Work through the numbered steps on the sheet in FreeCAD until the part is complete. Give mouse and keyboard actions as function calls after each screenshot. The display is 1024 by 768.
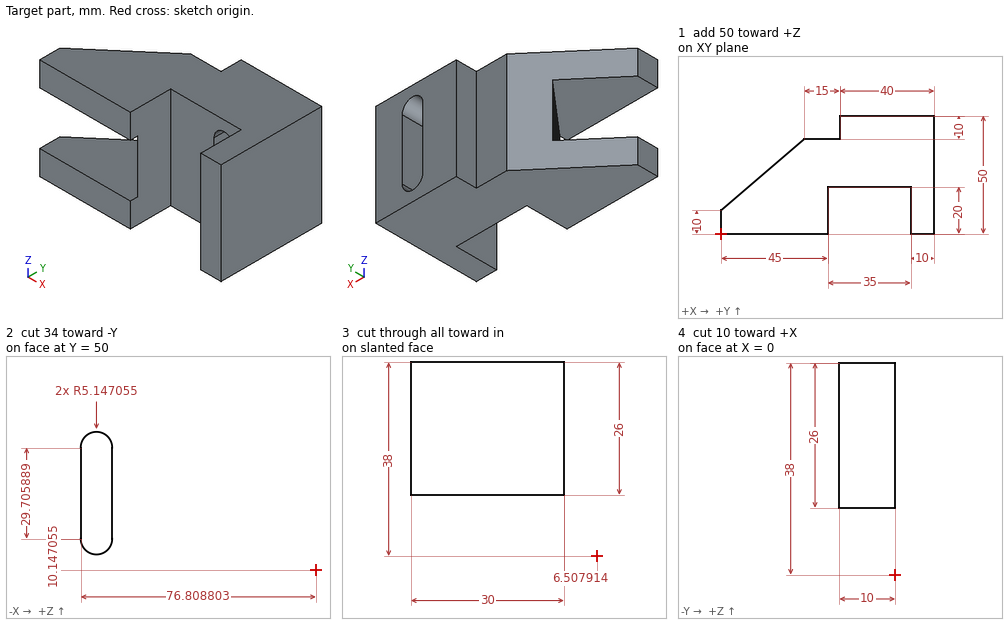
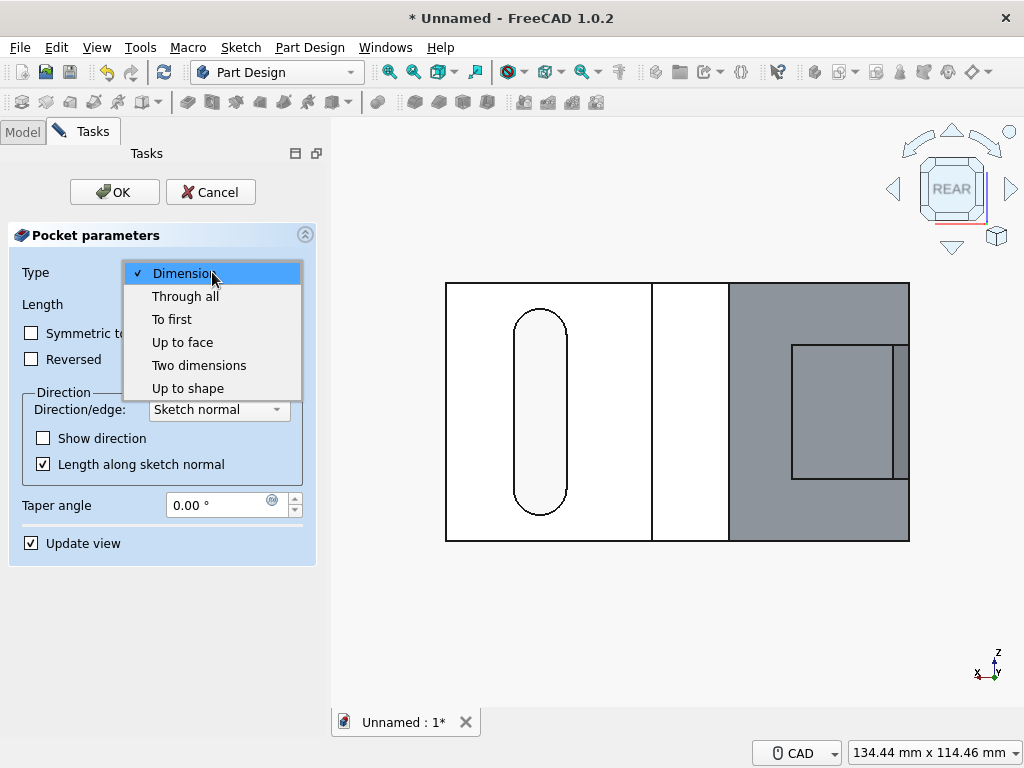
click(212, 296)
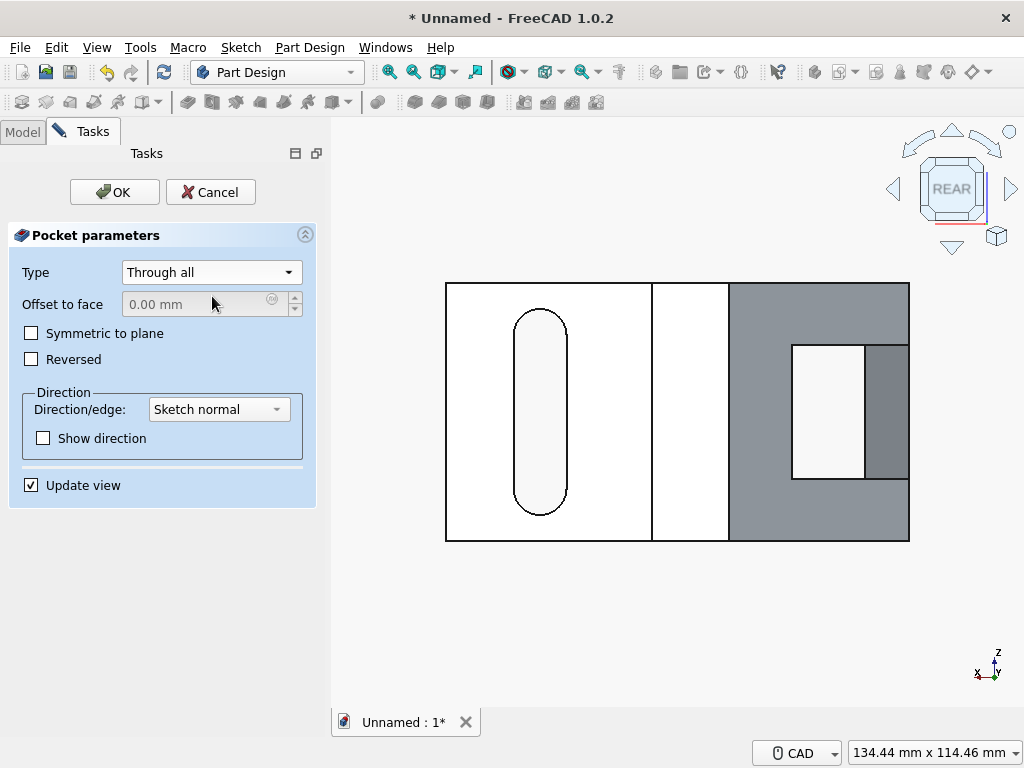
click(115, 192)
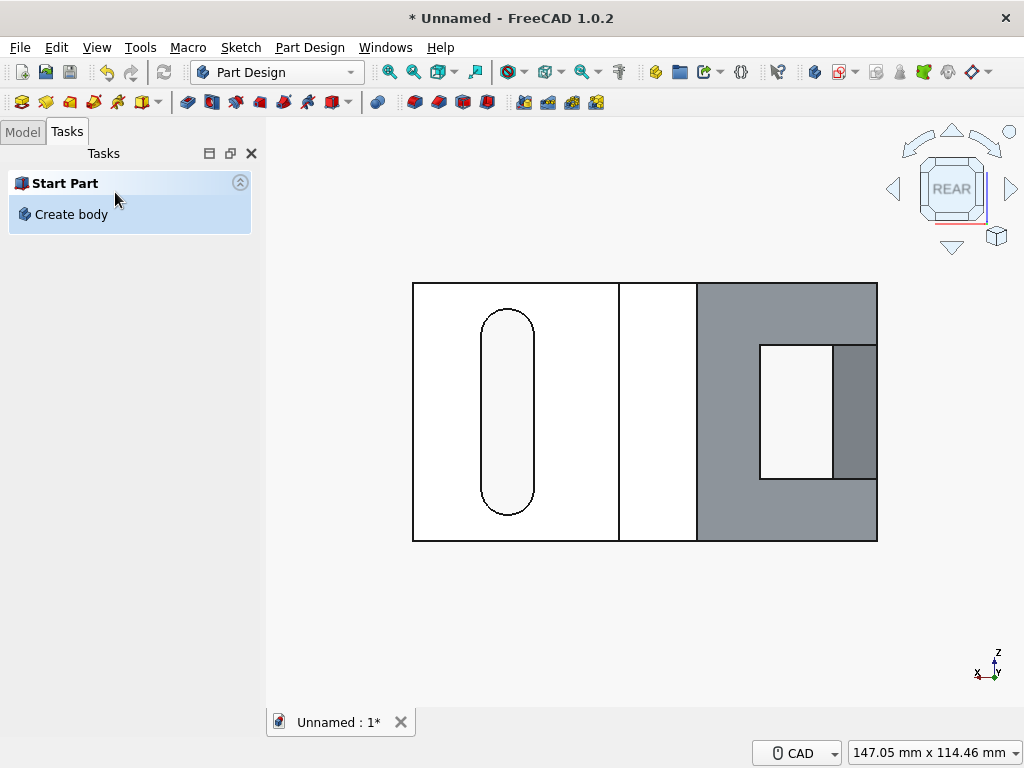
key(6)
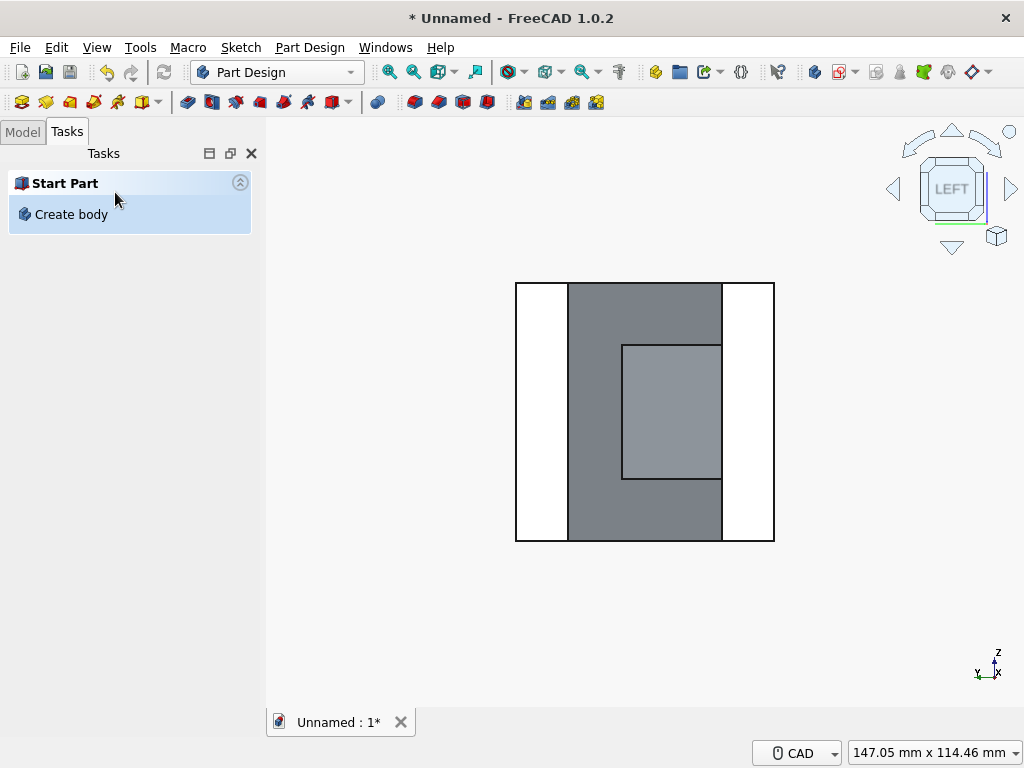
click(390, 72)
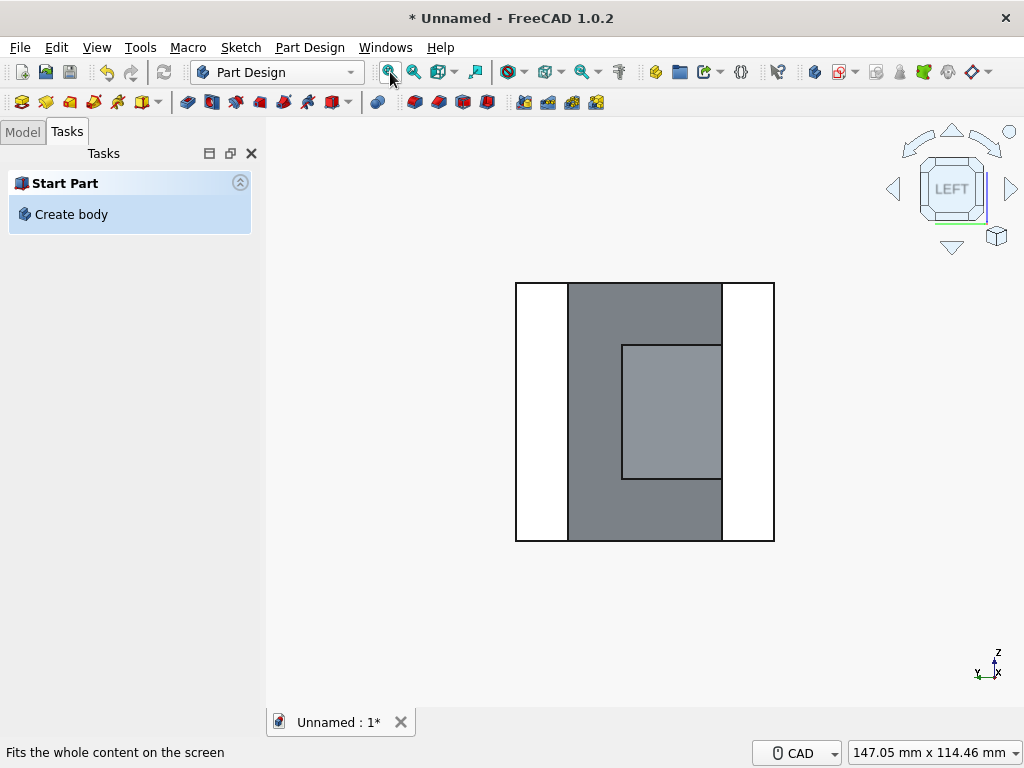
click(748, 337)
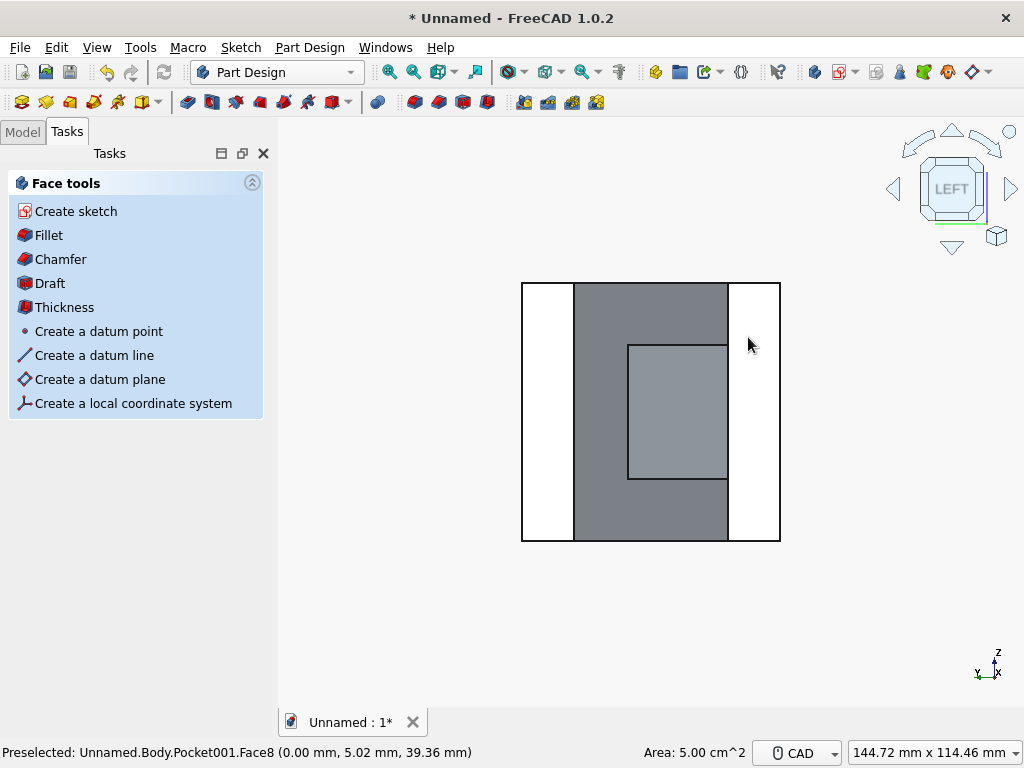
click(840, 72)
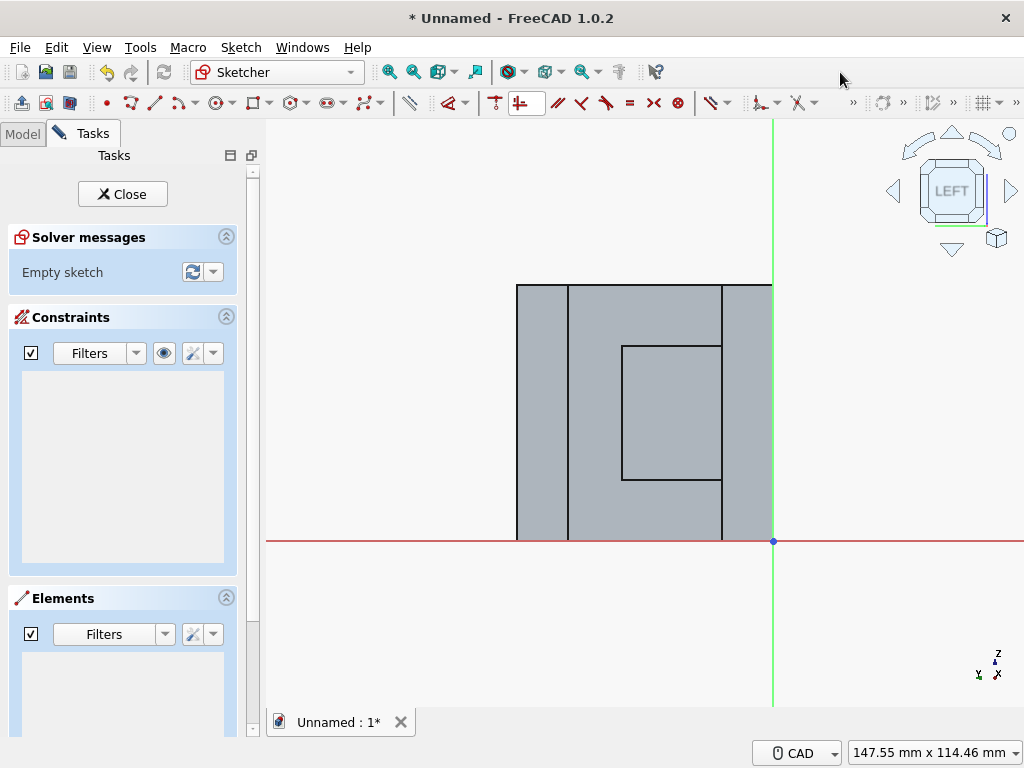
scroll(859, 481, up, 3)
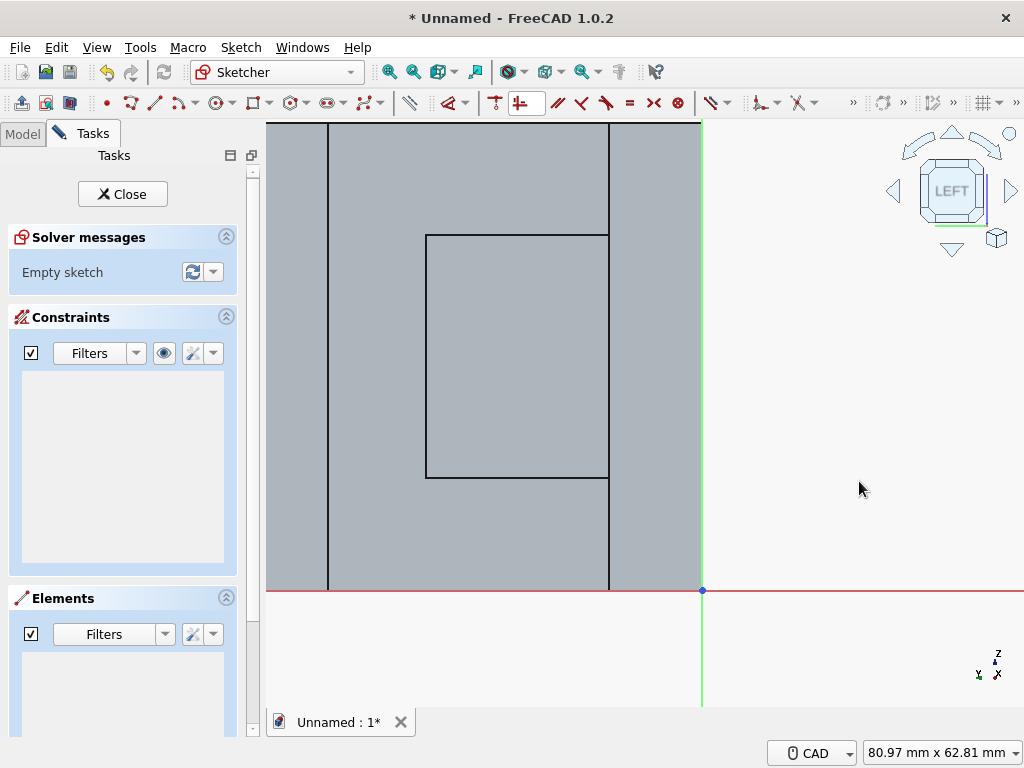
click(254, 104)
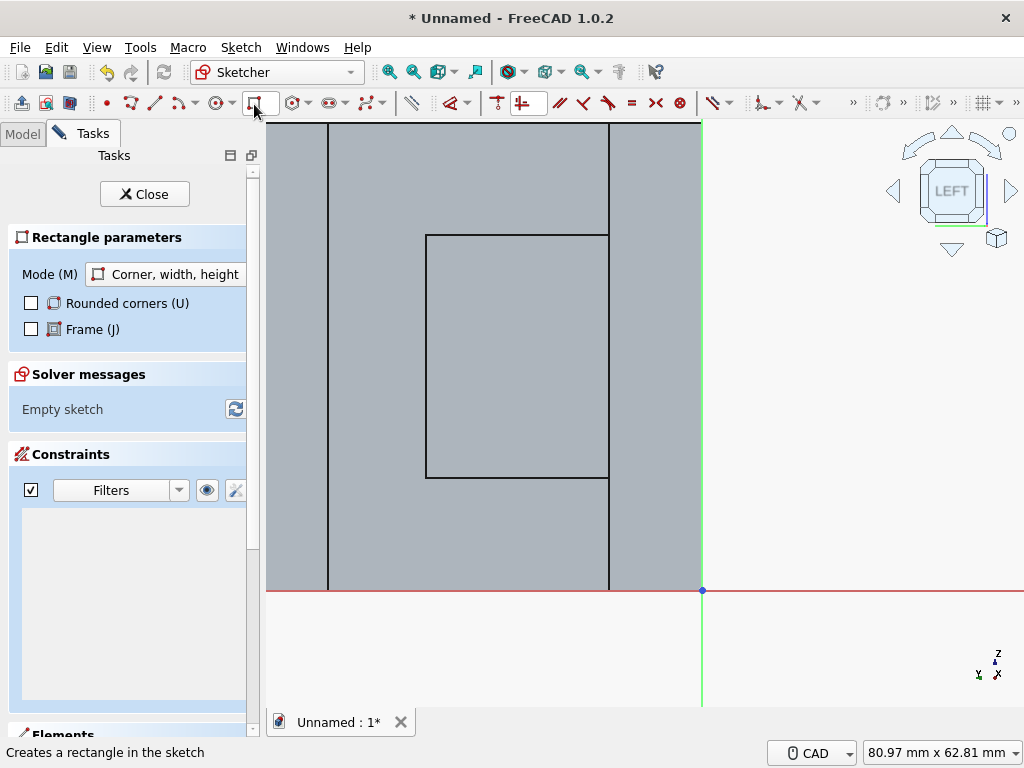
click(609, 235)
click(702, 478)
key(Escape)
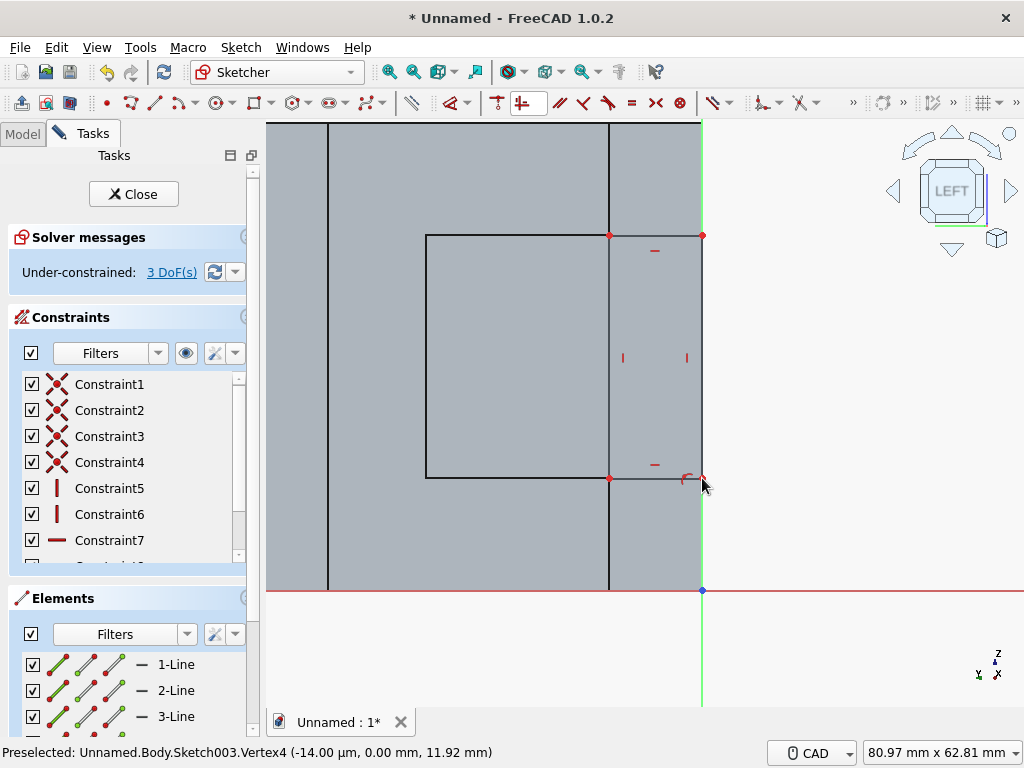
click(450, 104)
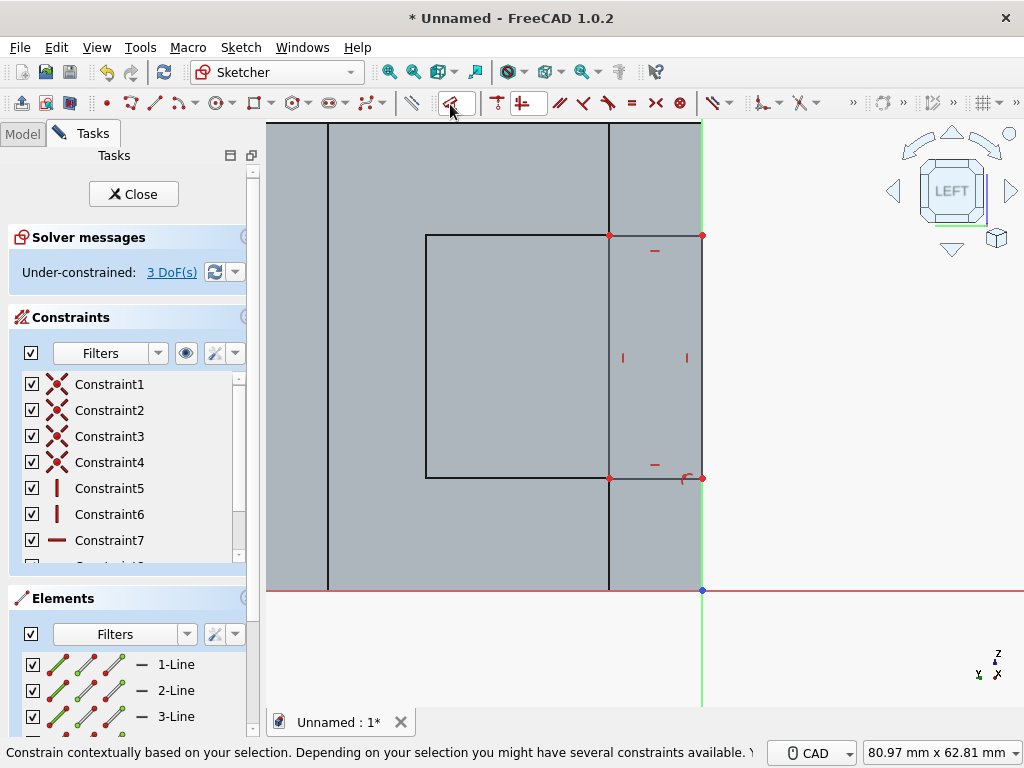
click(609, 309)
click(575, 358)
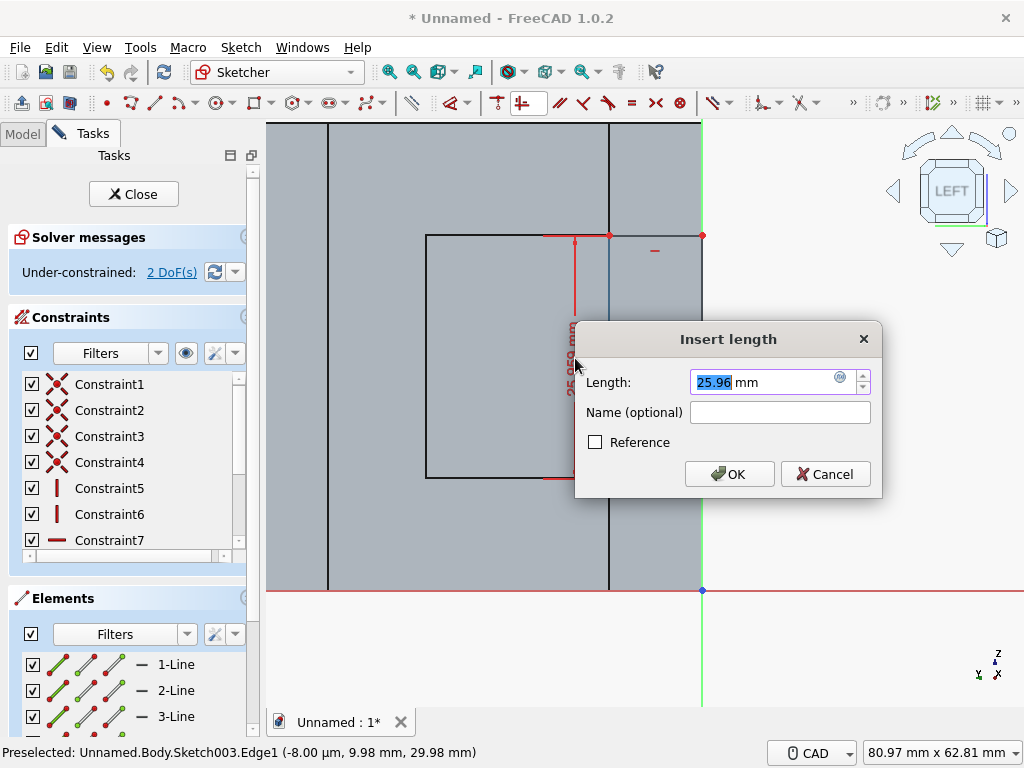
text(26)
key(Return)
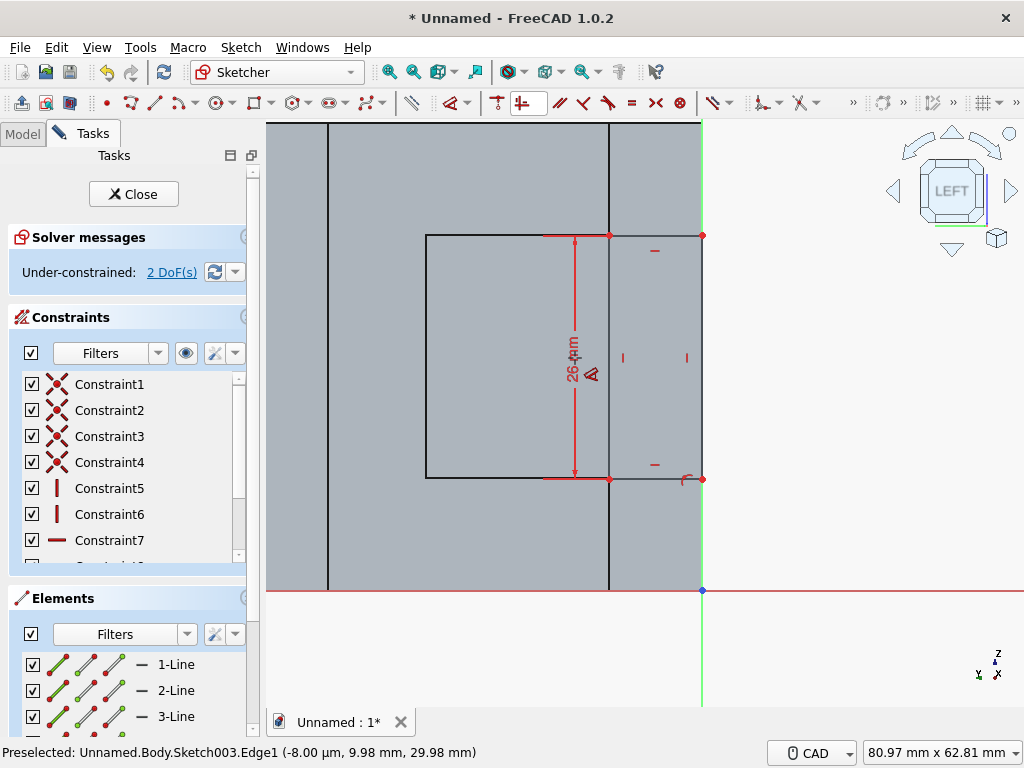
click(637, 479)
click(656, 513)